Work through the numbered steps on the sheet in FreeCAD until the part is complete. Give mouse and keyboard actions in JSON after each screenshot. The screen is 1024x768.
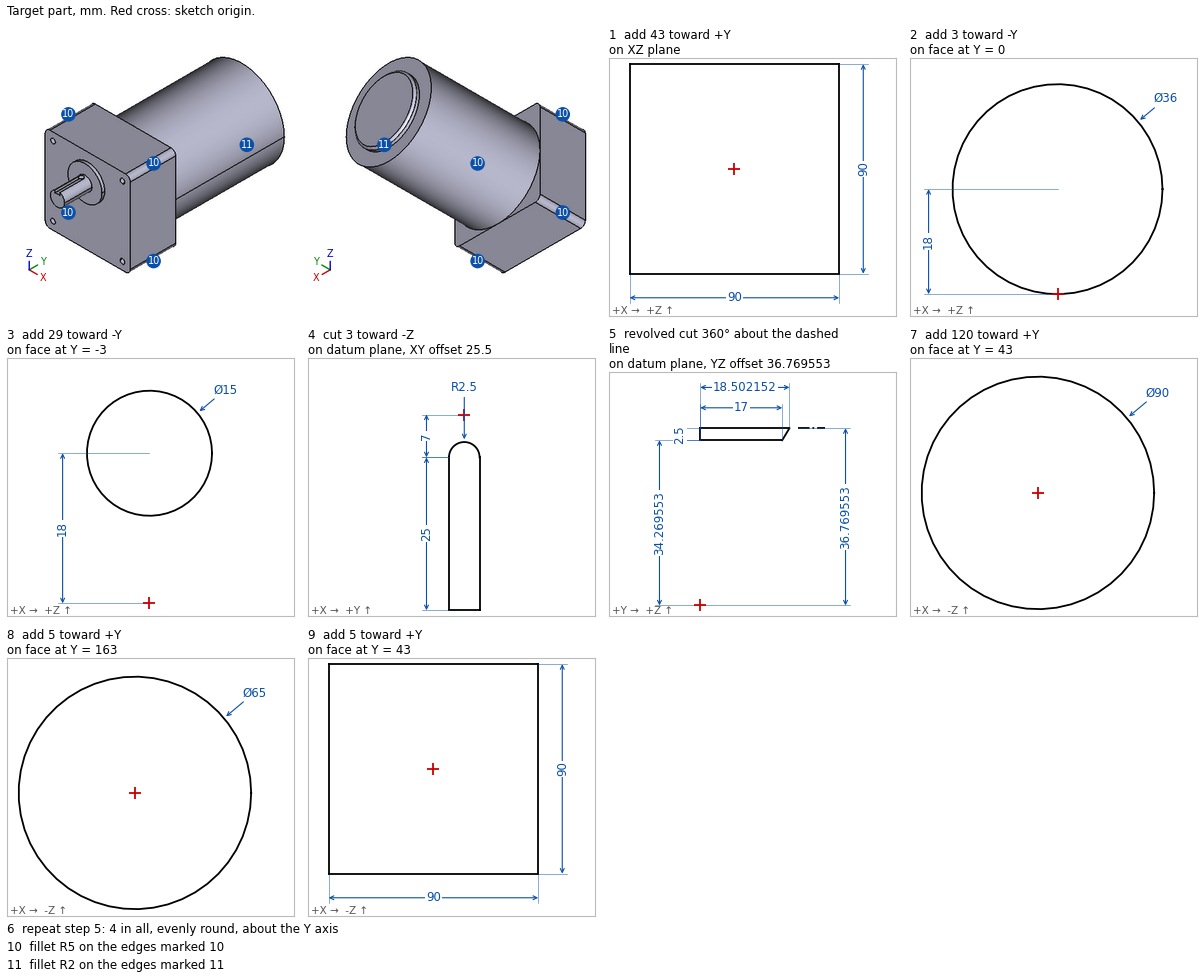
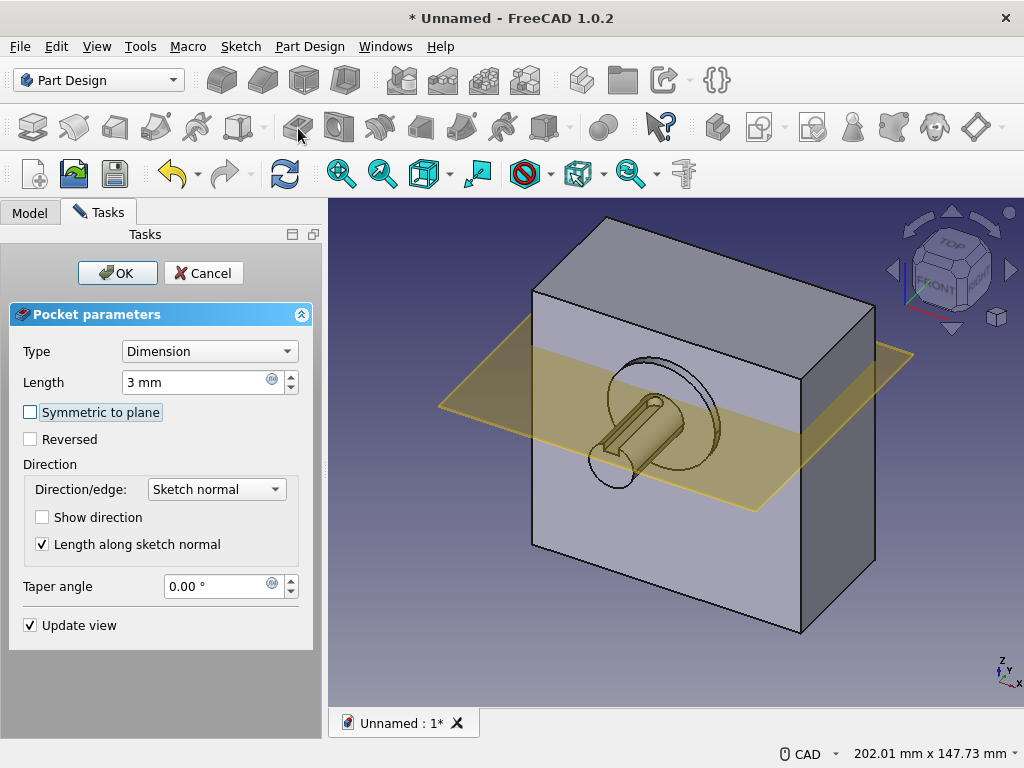
{"action": "left_click", "coordinate": [118, 273]}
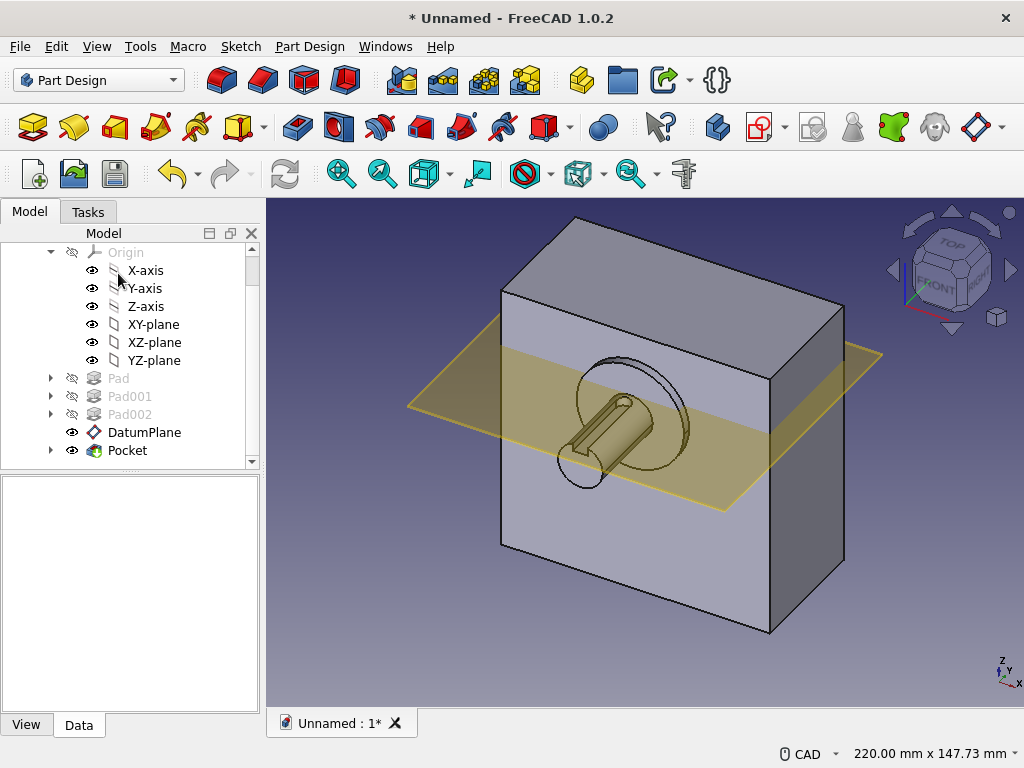
{"action": "left_click", "coordinate": [117, 432]}
{"action": "key", "text": "space"}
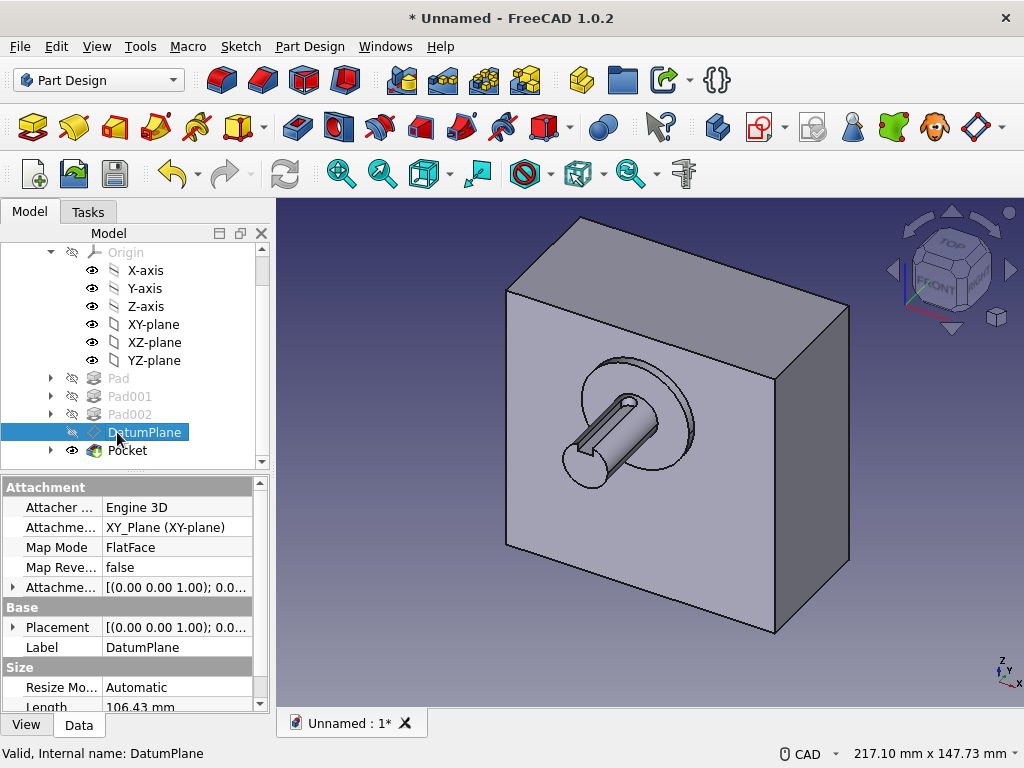
{"action": "left_click", "coordinate": [137, 360]}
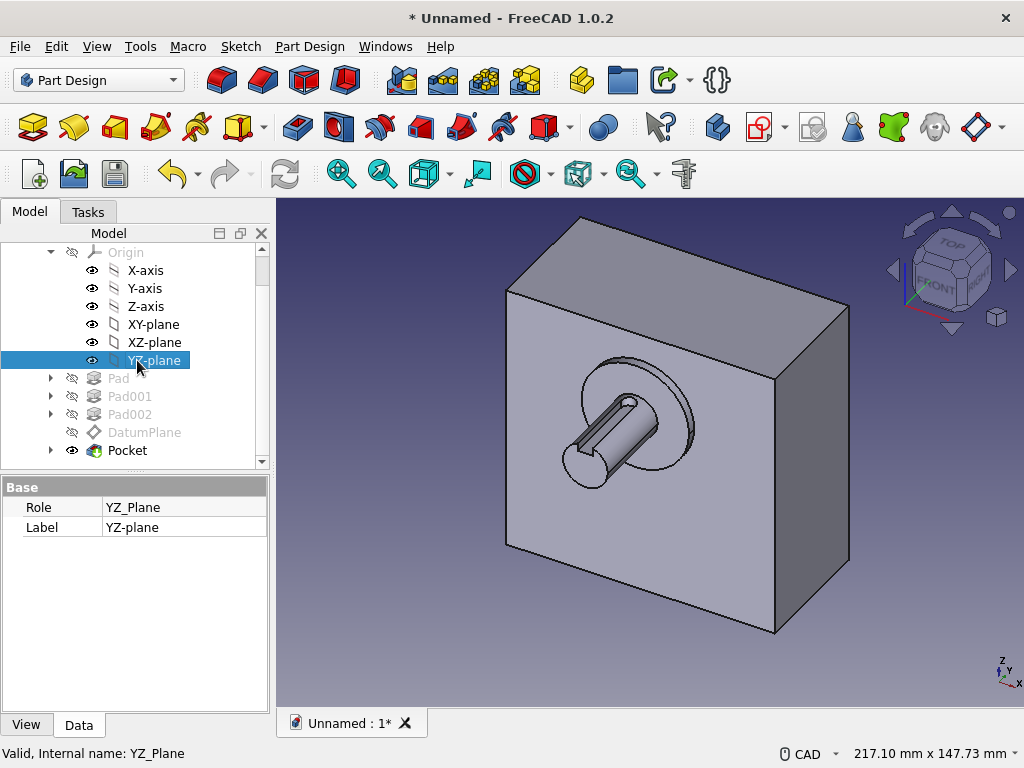
{"action": "left_click", "coordinate": [976, 128]}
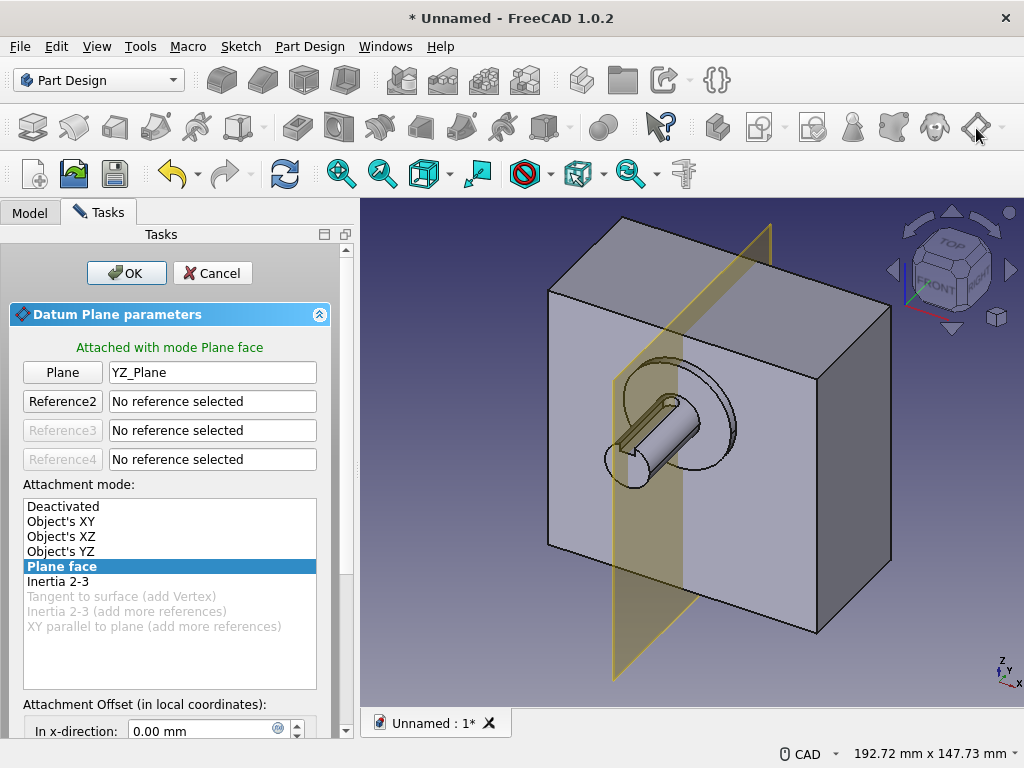
{"action": "scroll", "coordinate": [346, 491], "scroll_direction": "down", "scroll_amount": 3}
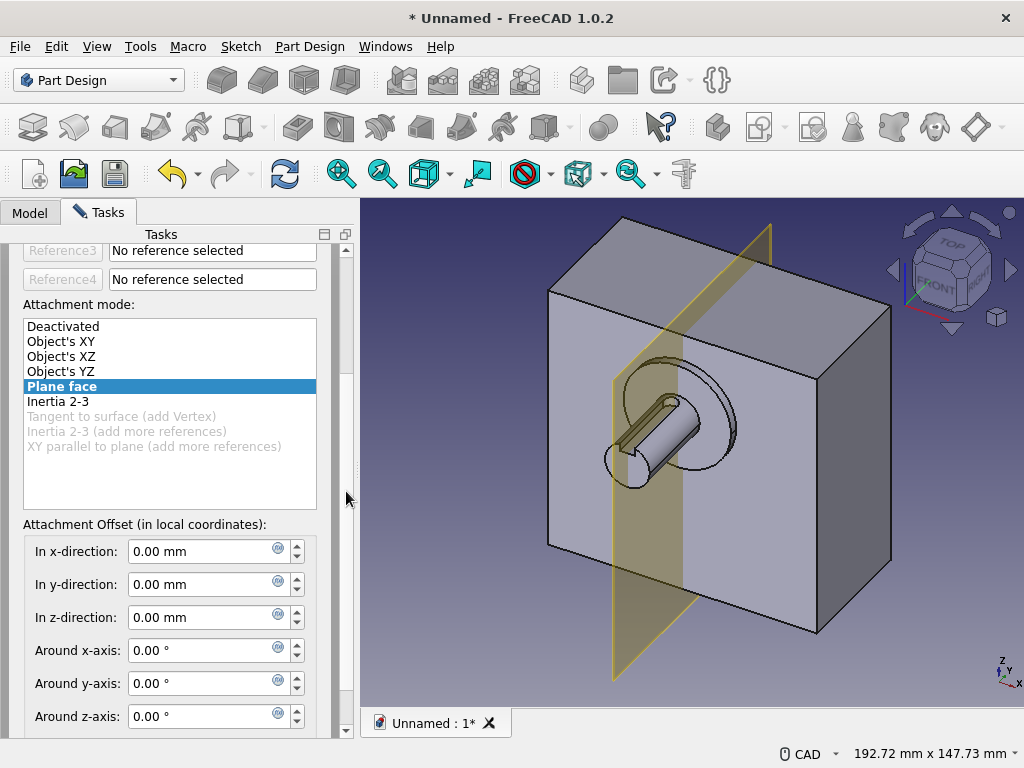
{"action": "triple_click", "coordinate": [210, 618]}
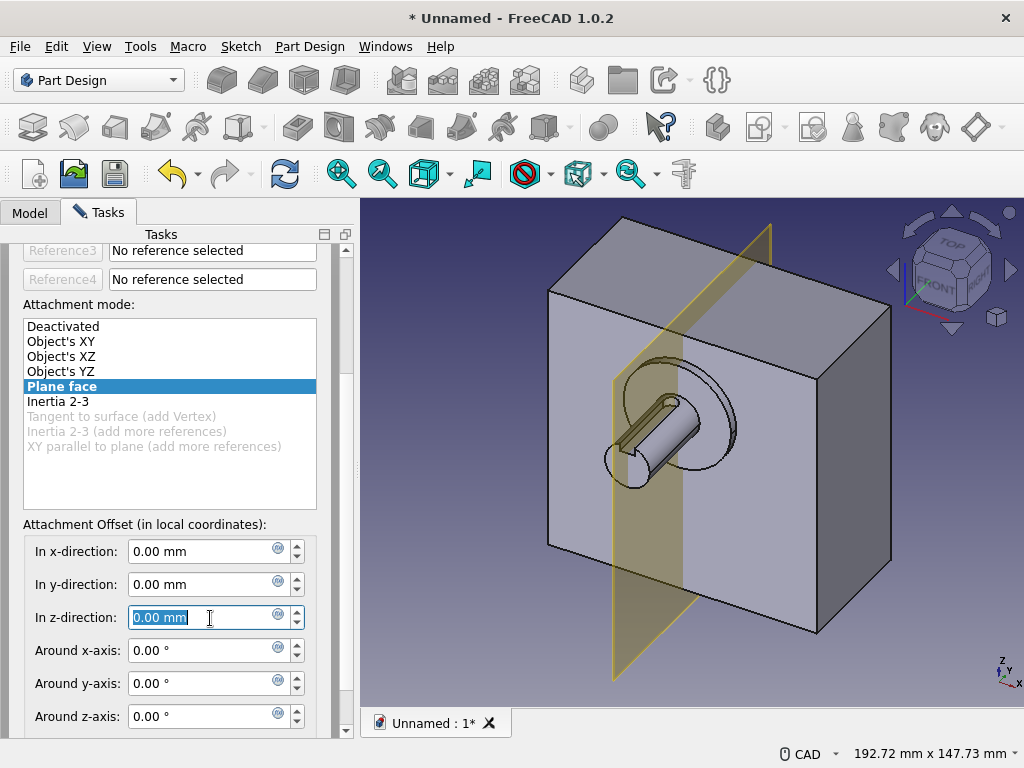
{"action": "type", "text": "36.769553"}
{"action": "key", "text": "Tab"}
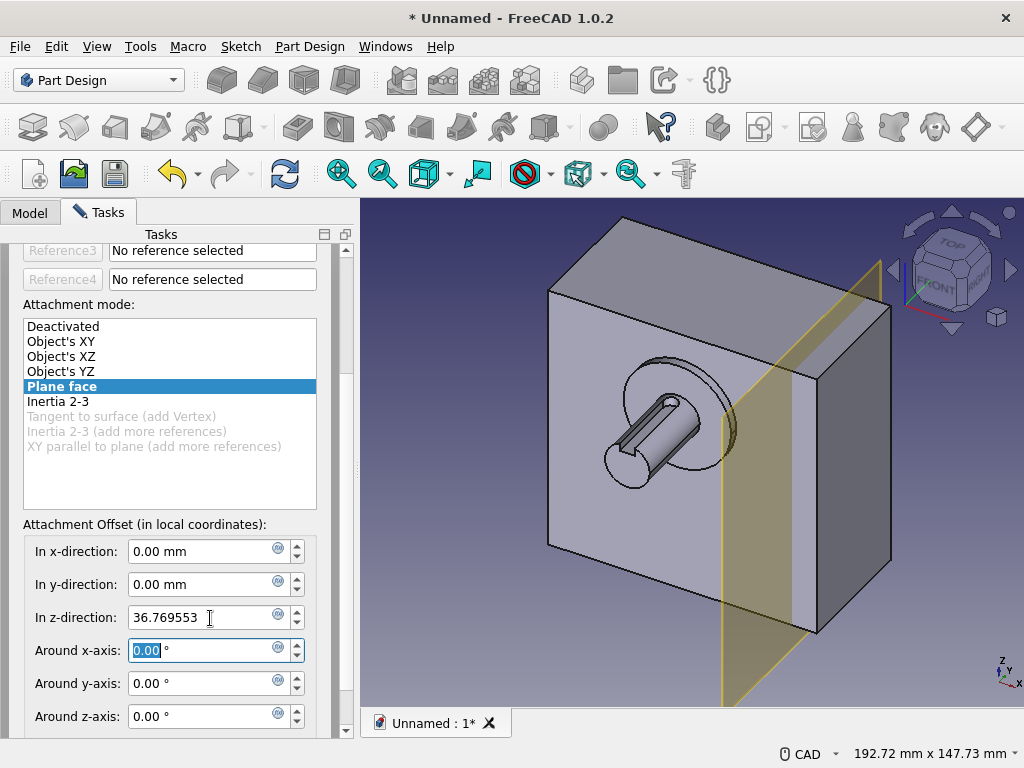
{"action": "scroll", "coordinate": [346, 491], "scroll_direction": "up", "scroll_amount": 4}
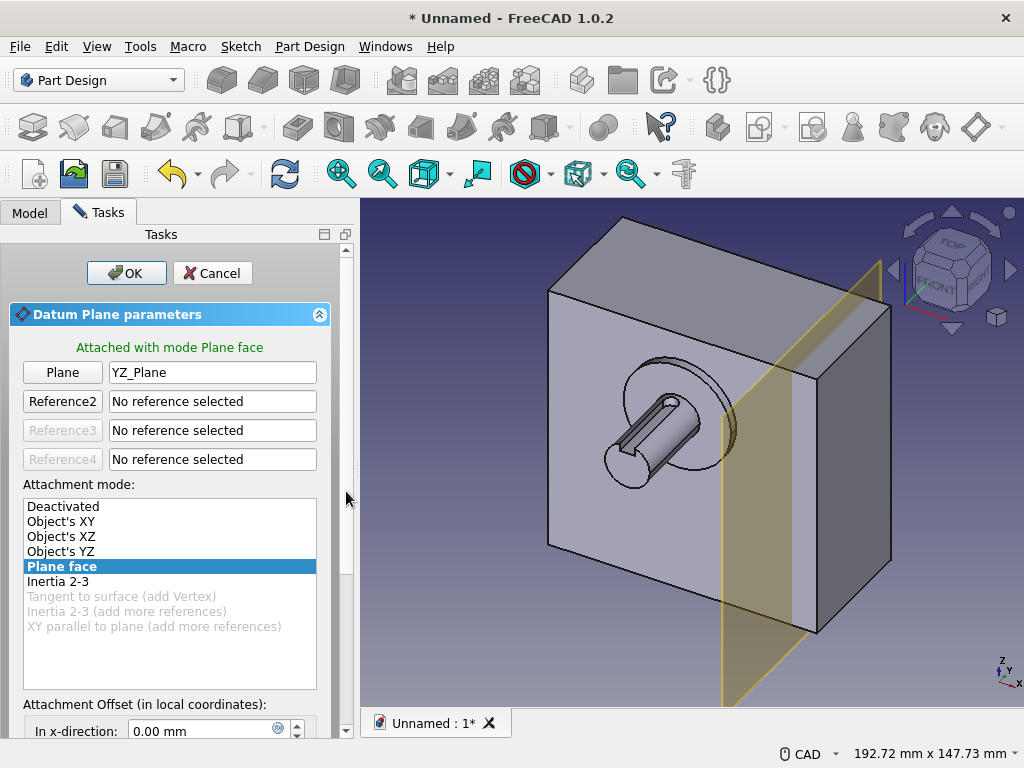
{"action": "left_click", "coordinate": [127, 273]}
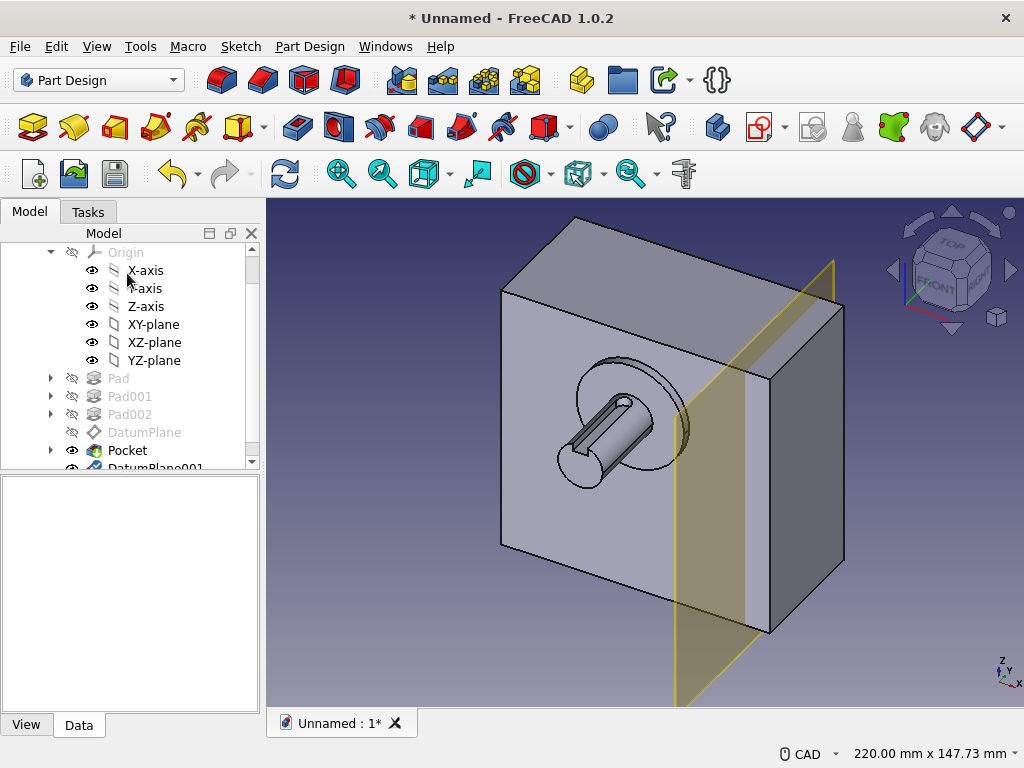
{"action": "left_click", "coordinate": [117, 468]}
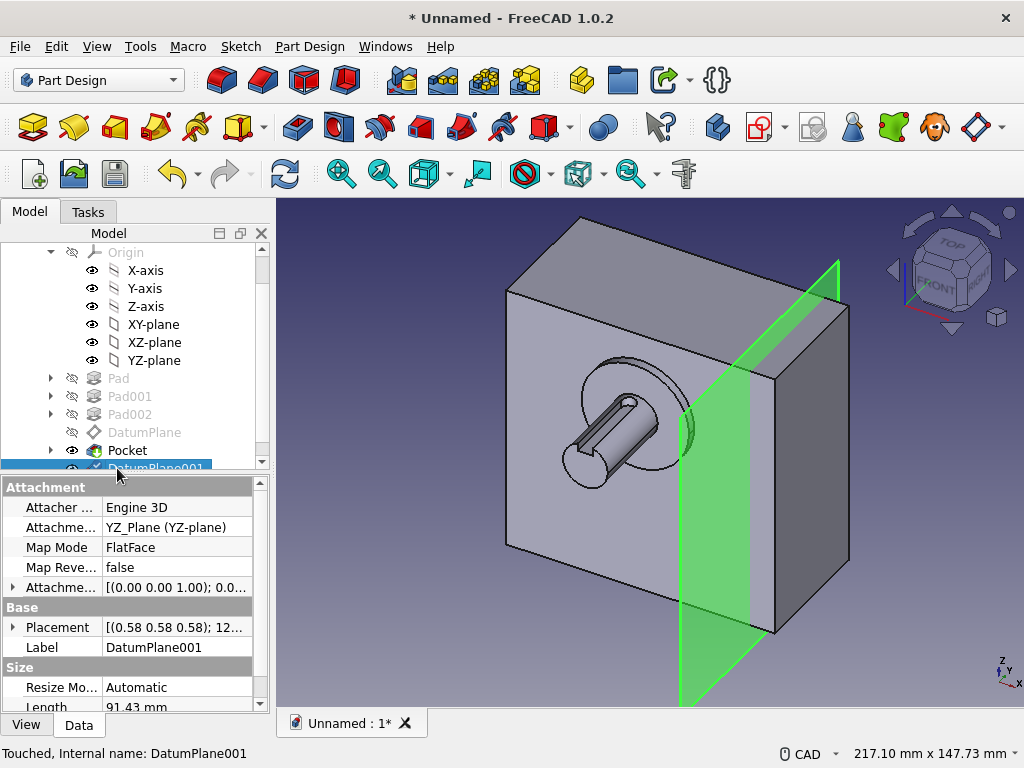
{"action": "left_click", "coordinate": [758, 128]}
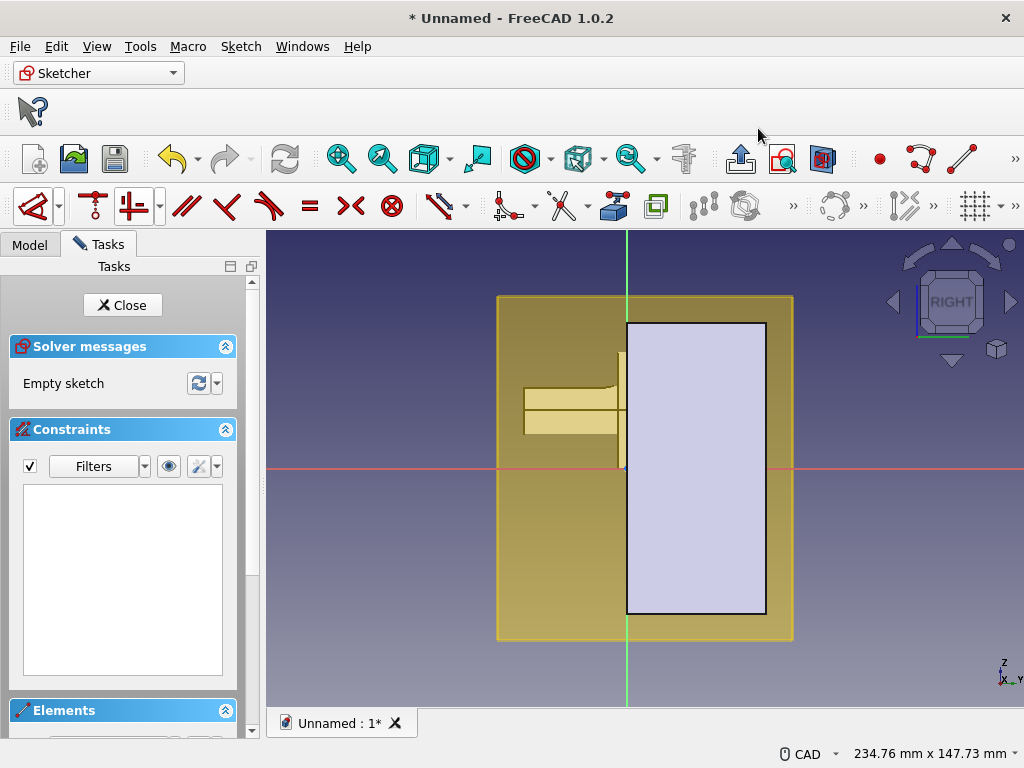
{"action": "left_click", "coordinate": [823, 160]}